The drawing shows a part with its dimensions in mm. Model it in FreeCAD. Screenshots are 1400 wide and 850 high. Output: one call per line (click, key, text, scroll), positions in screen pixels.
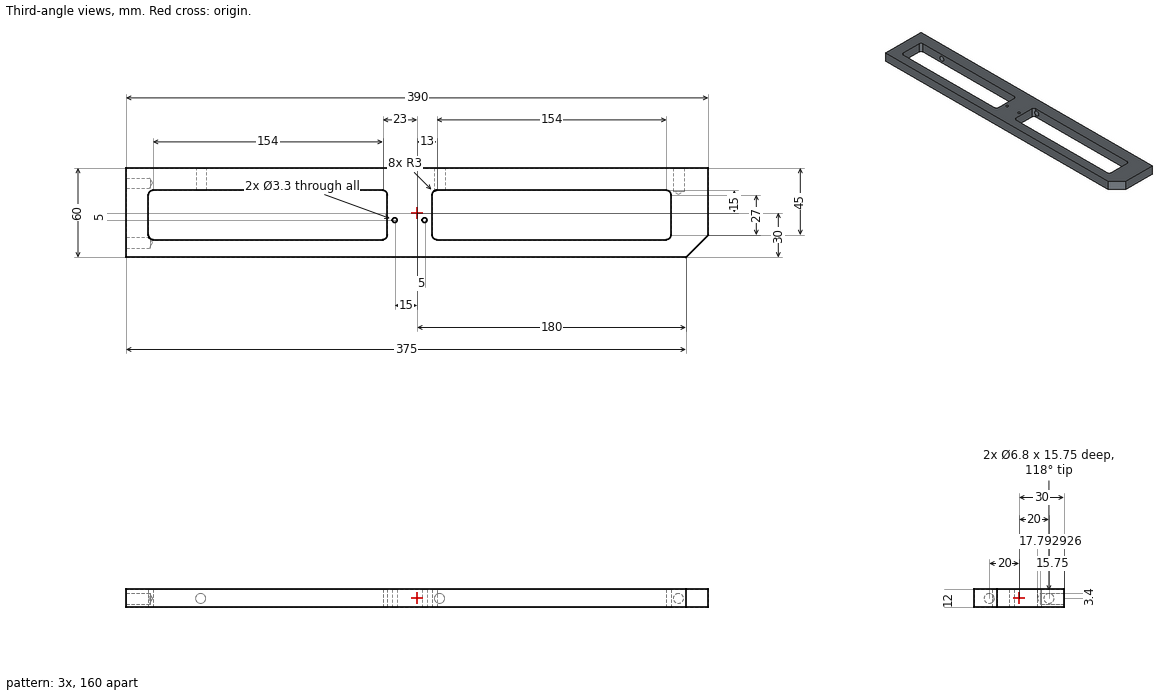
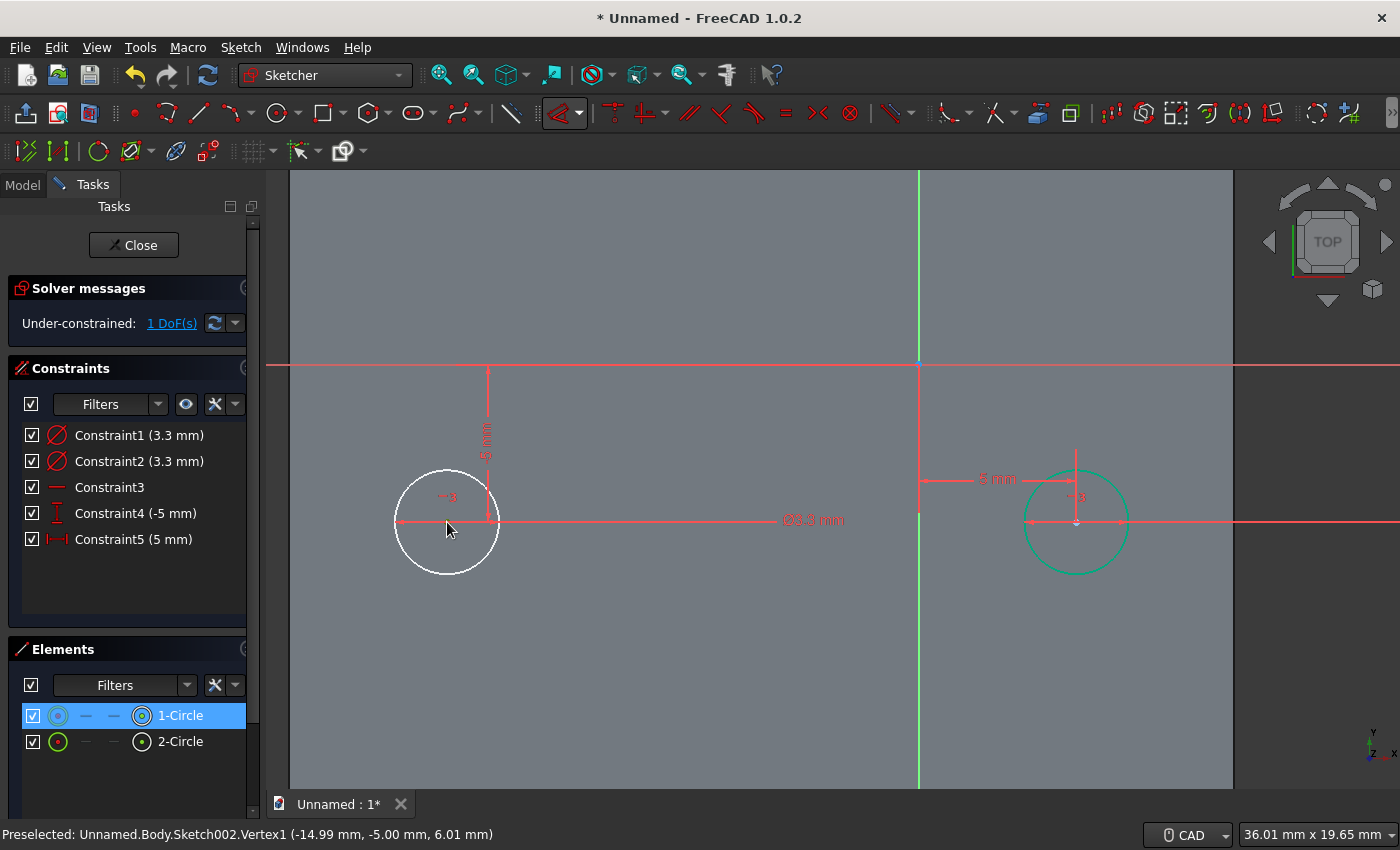
click(582, 114)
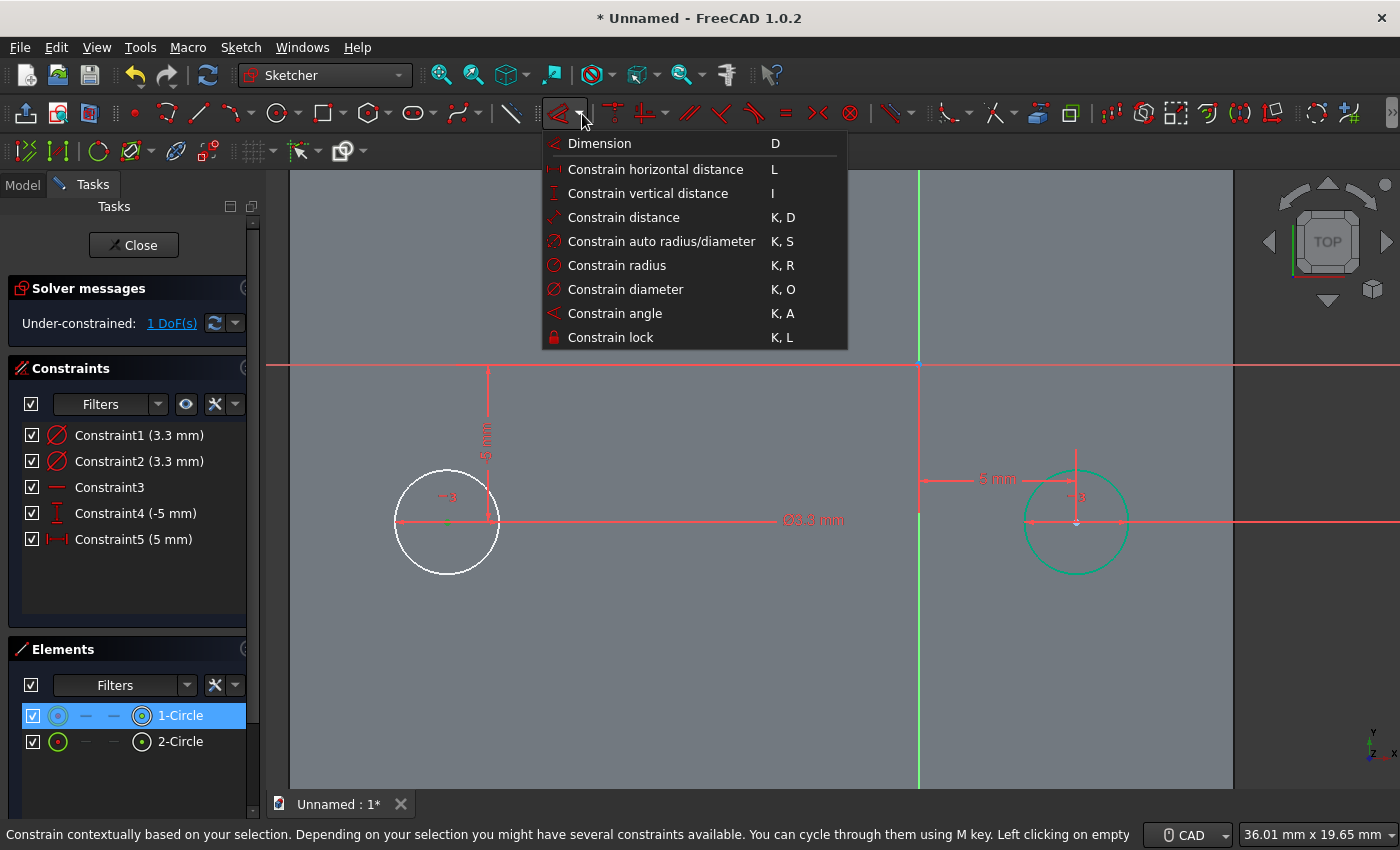
click(695, 169)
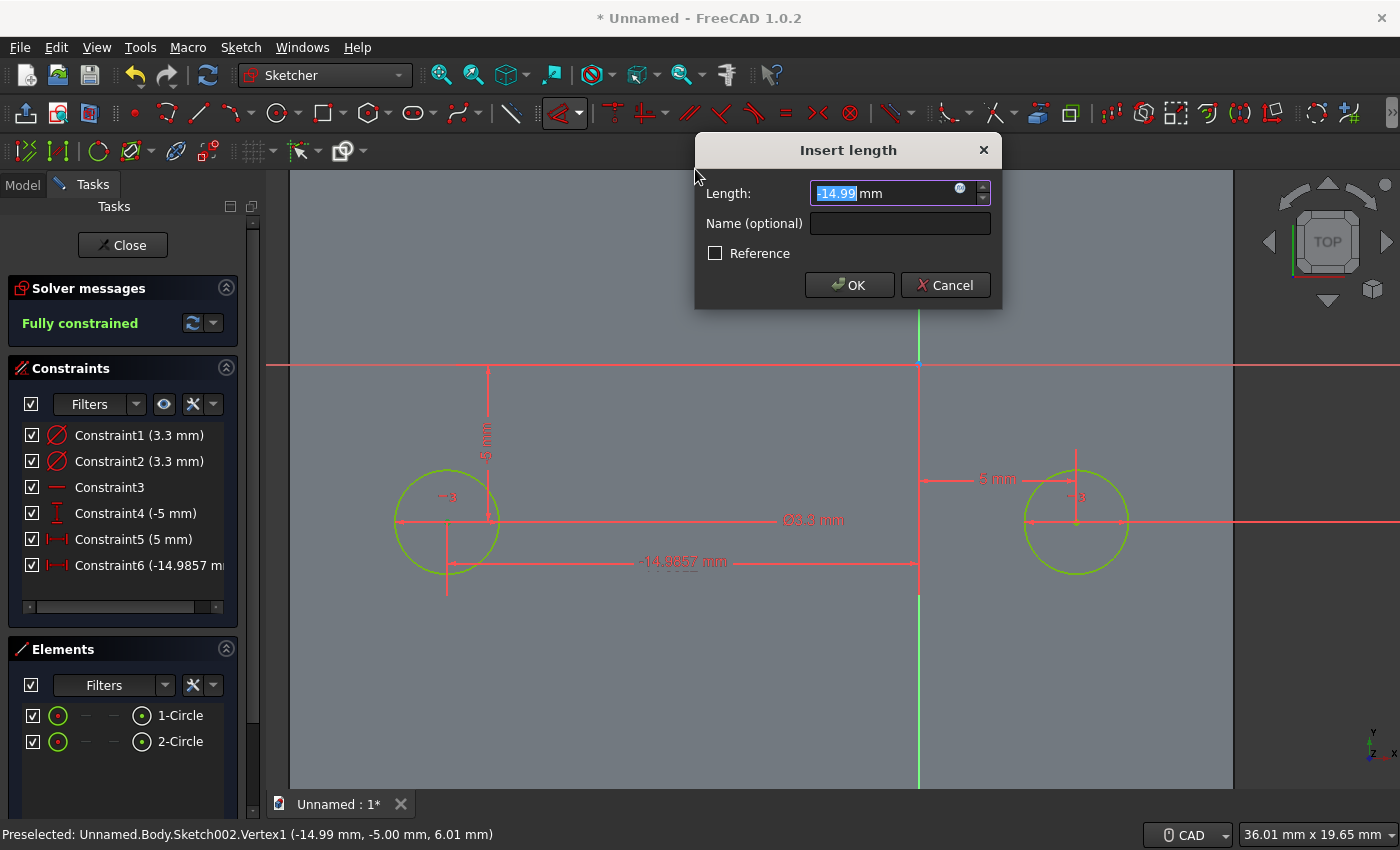
text(-15)
key(Return)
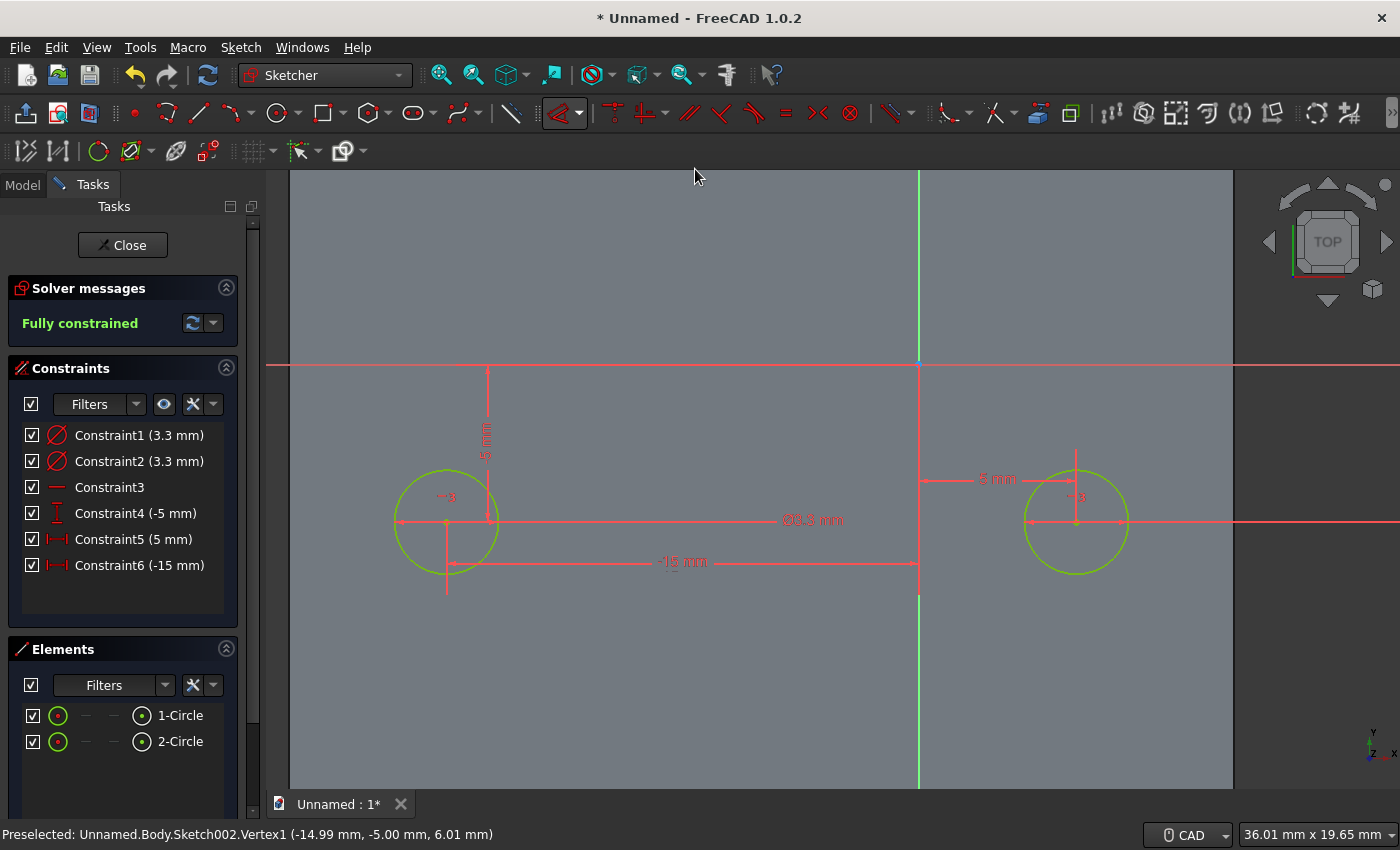
click(123, 245)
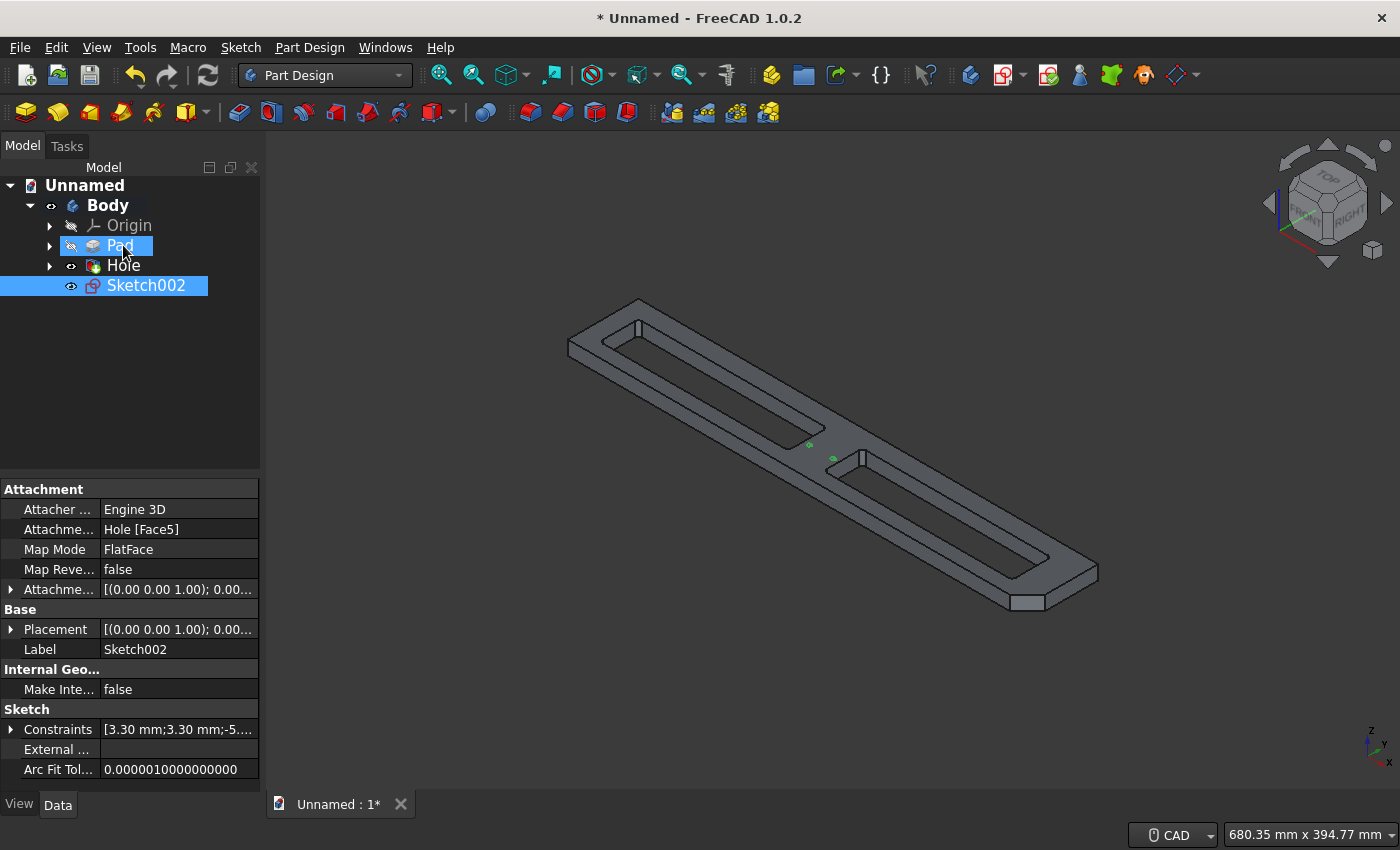
click(272, 112)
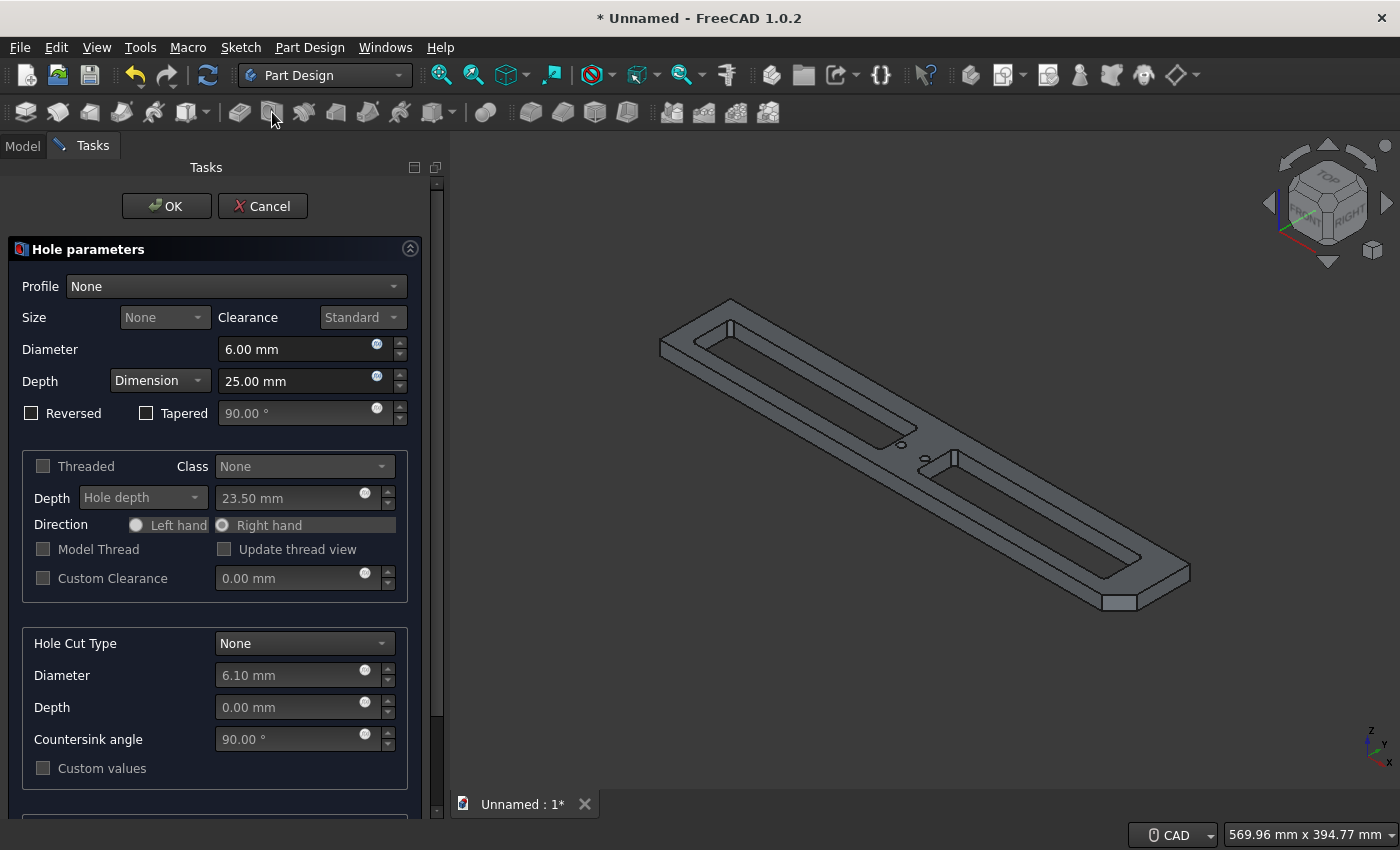
triple_click(305, 349)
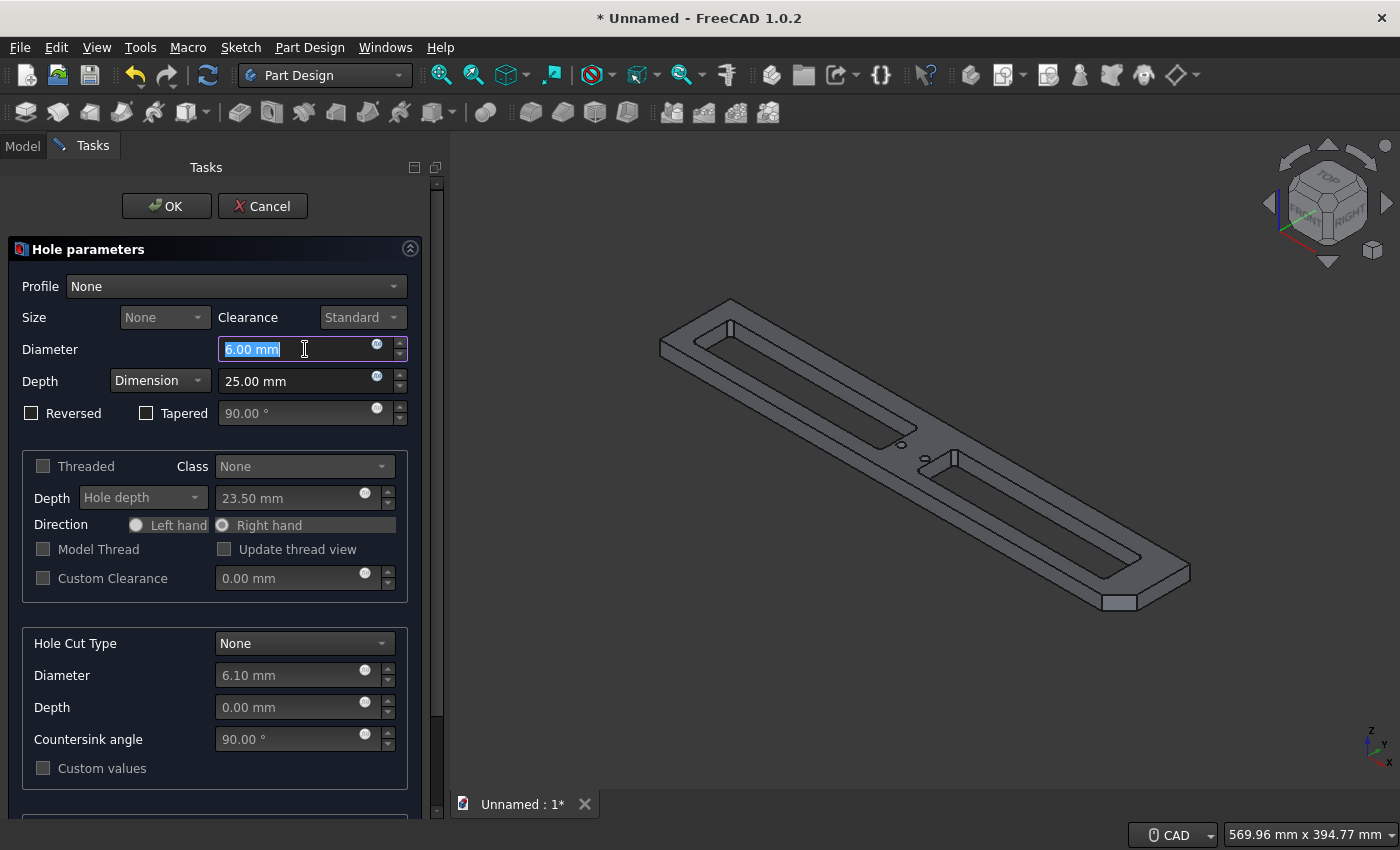
text(3.3)
key(Tab)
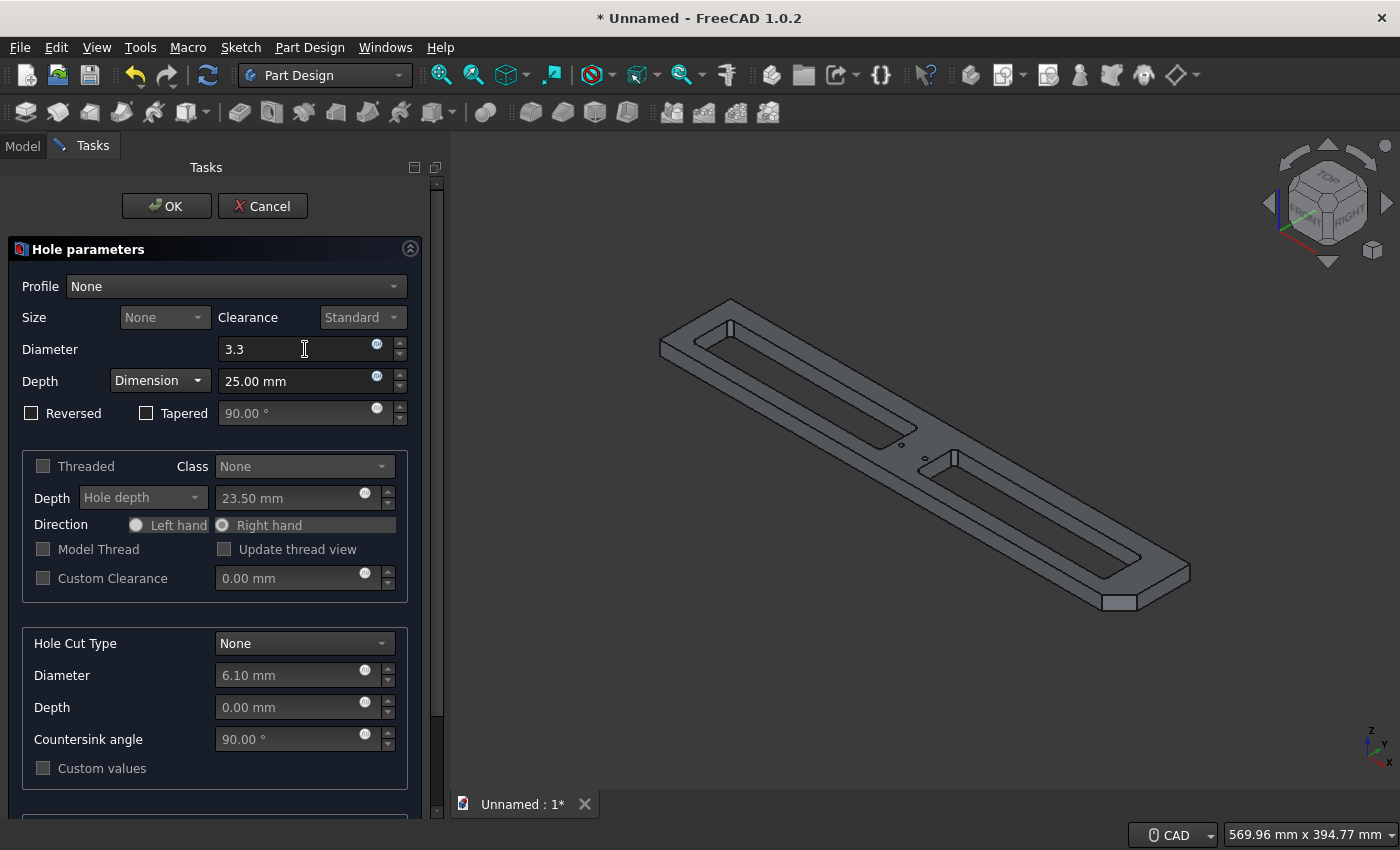
click(161, 380)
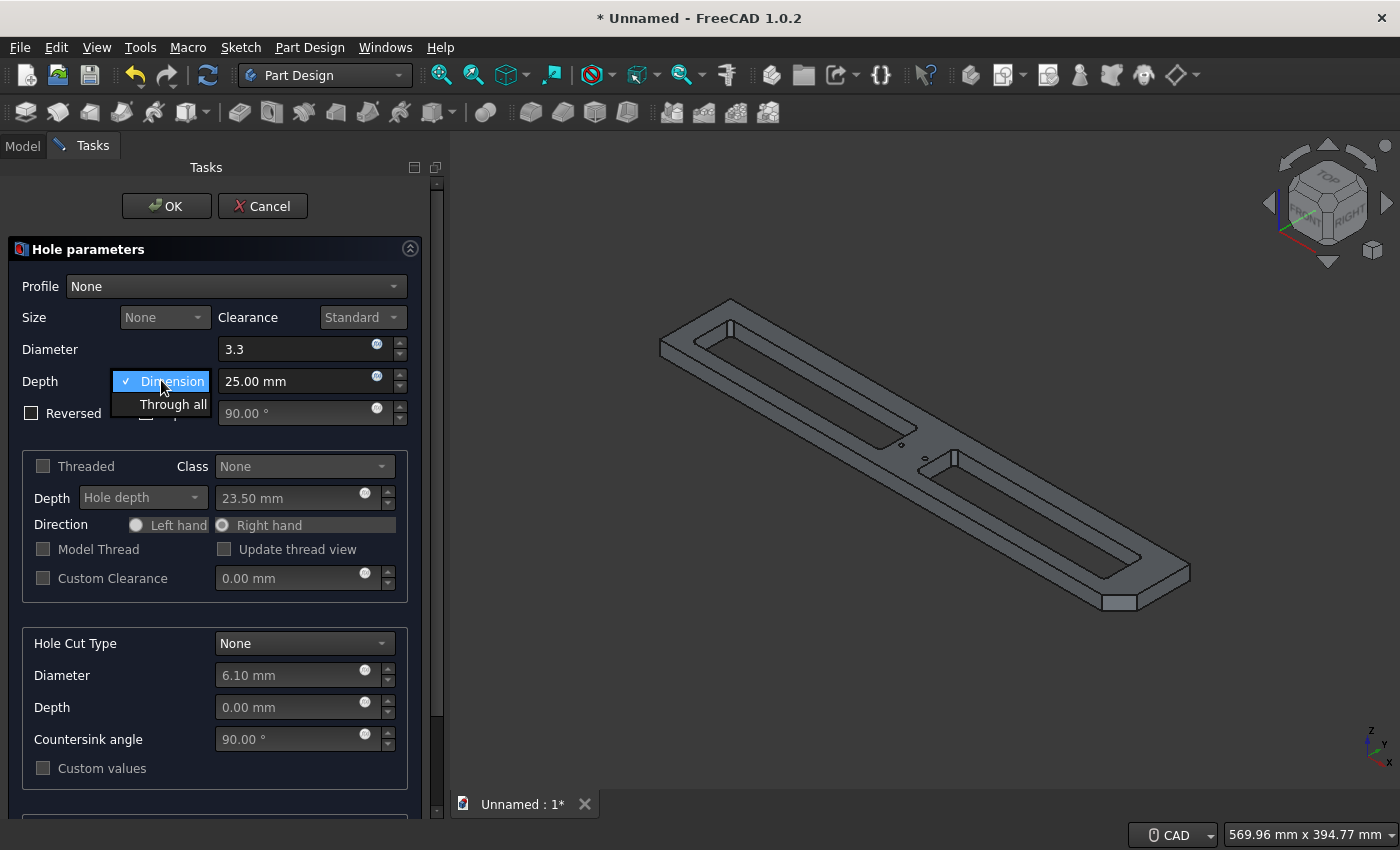
click(160, 404)